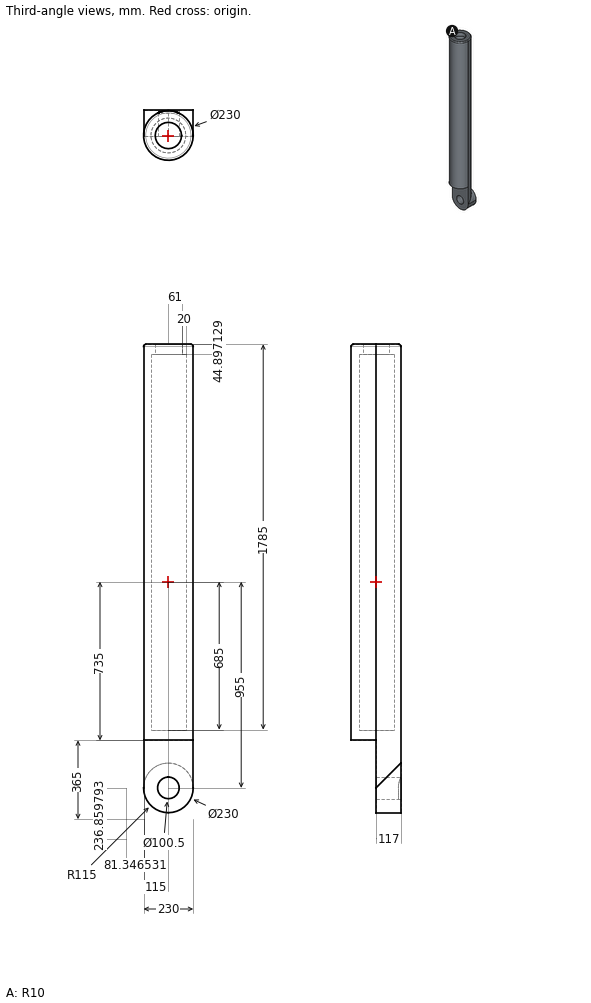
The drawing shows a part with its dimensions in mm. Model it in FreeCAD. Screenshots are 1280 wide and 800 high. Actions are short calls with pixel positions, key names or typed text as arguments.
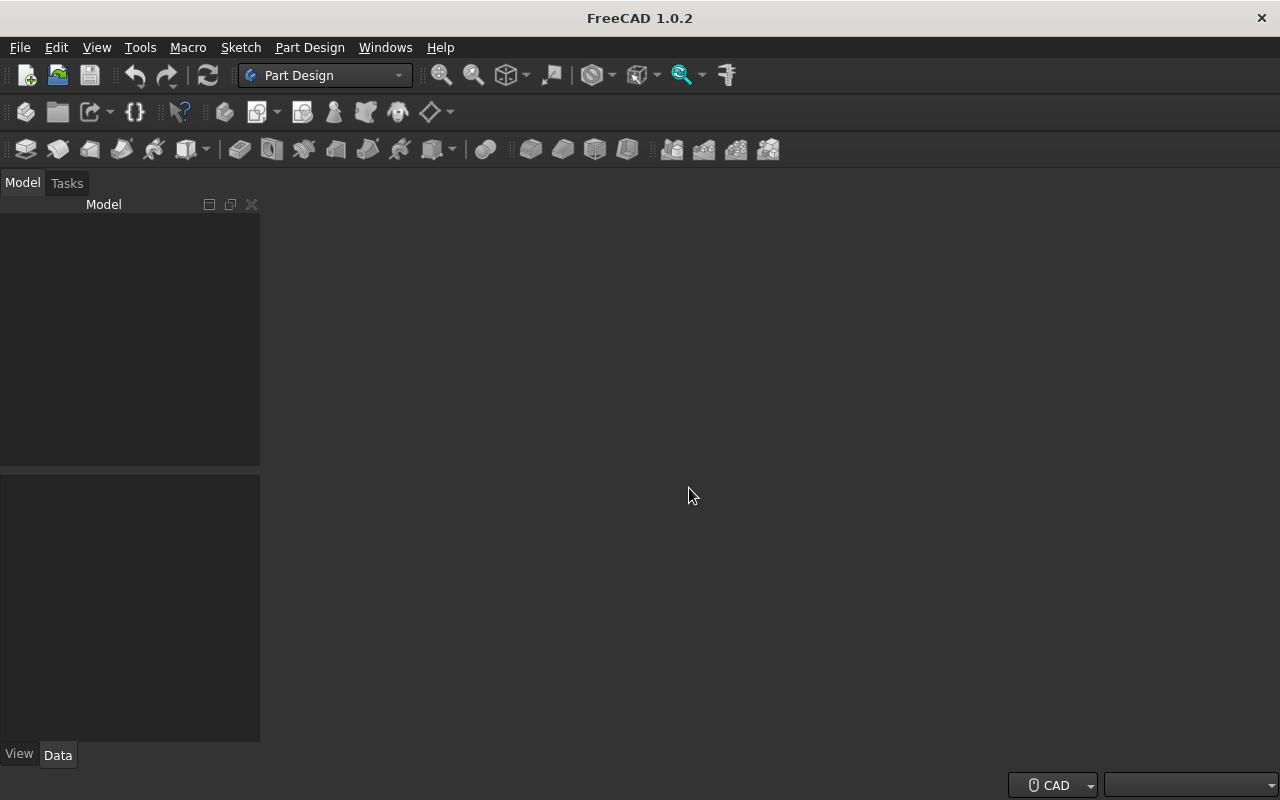
click(26, 76)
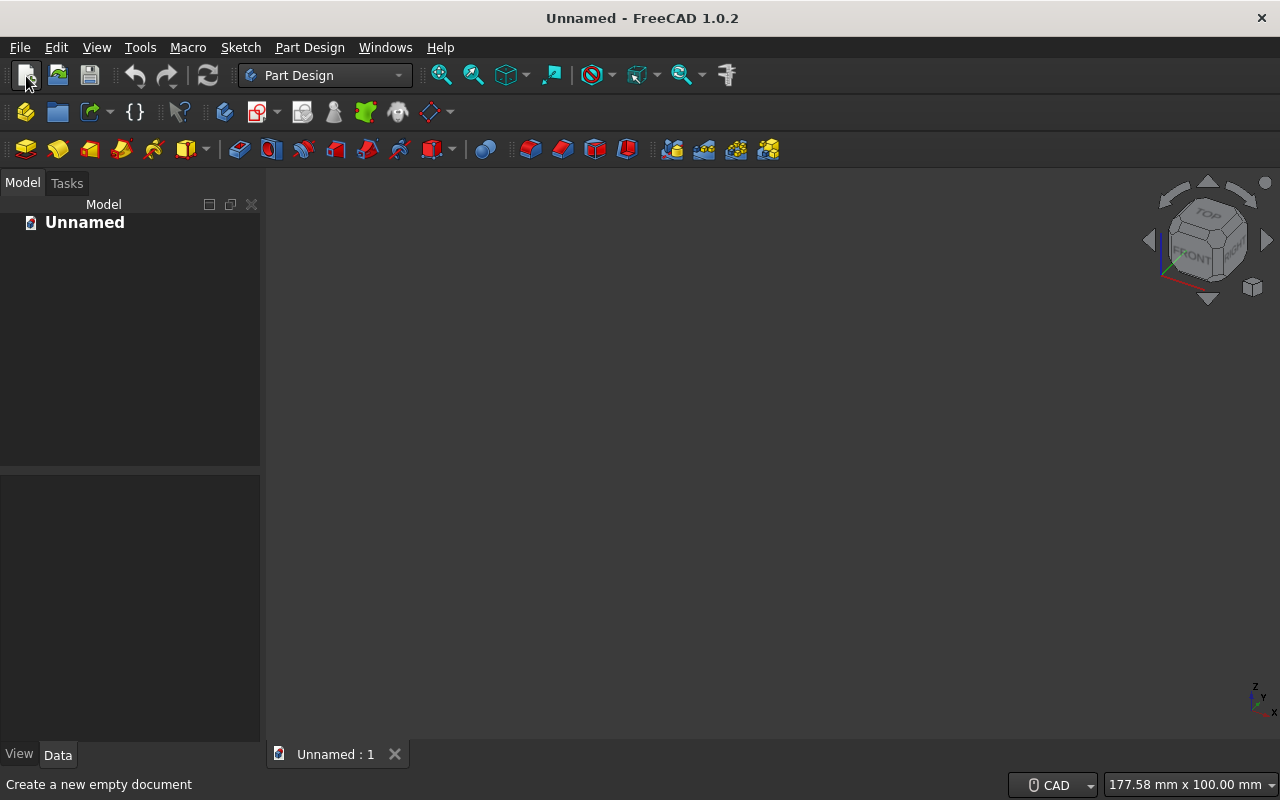
click(258, 112)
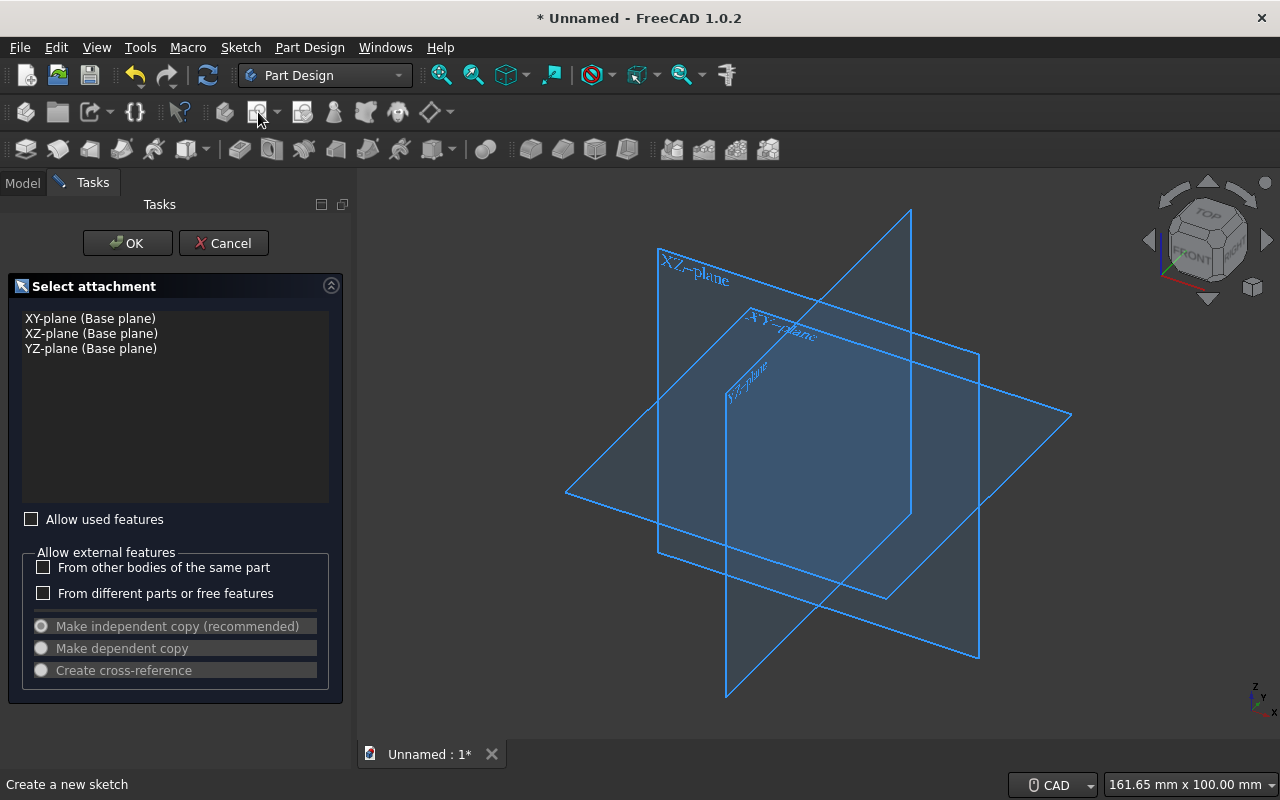
click(82, 318)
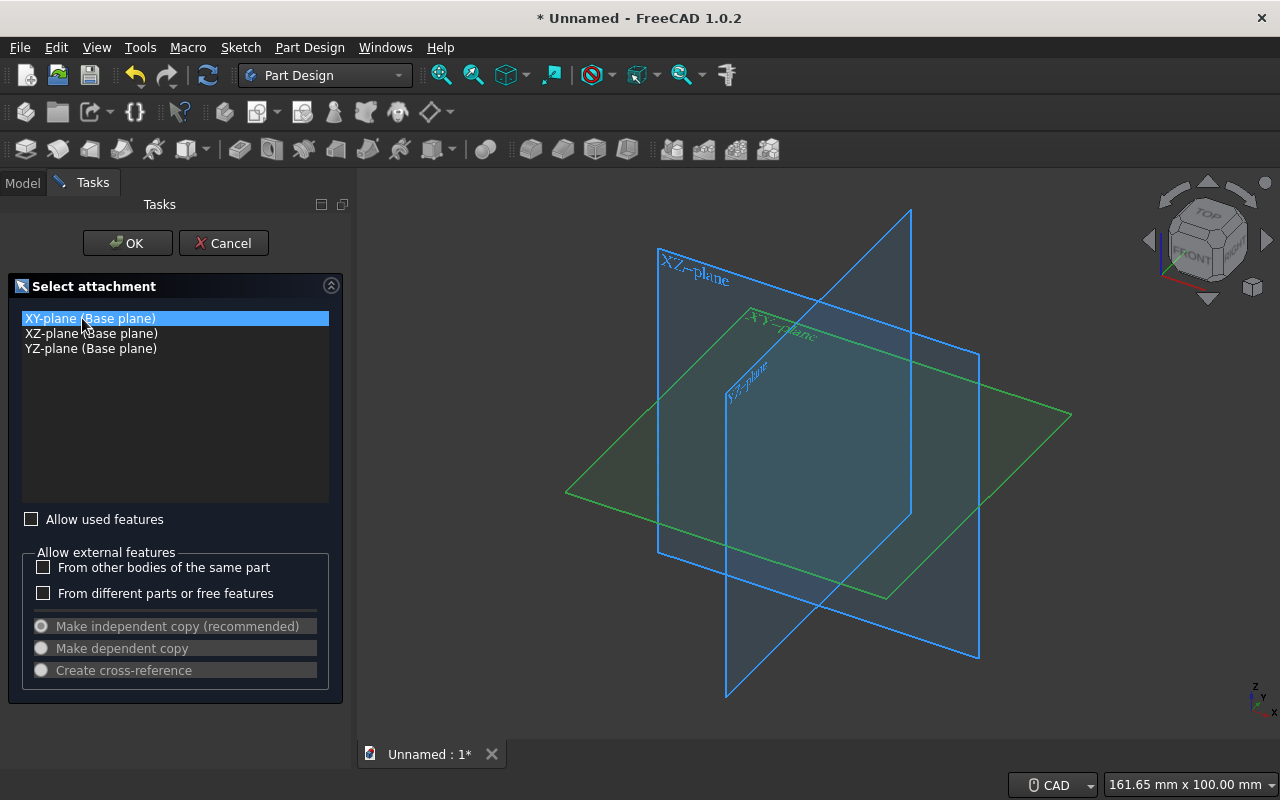
click(128, 243)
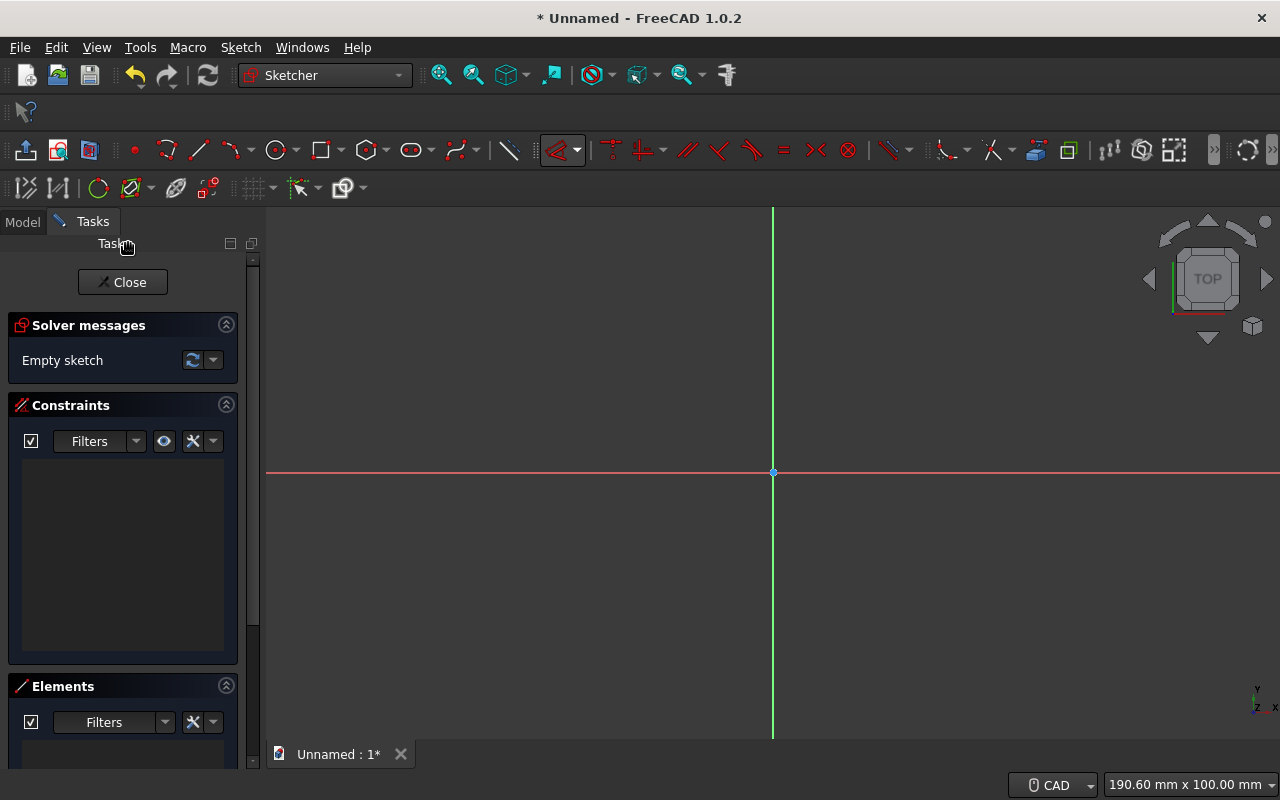
scroll(675, 473, down, 6)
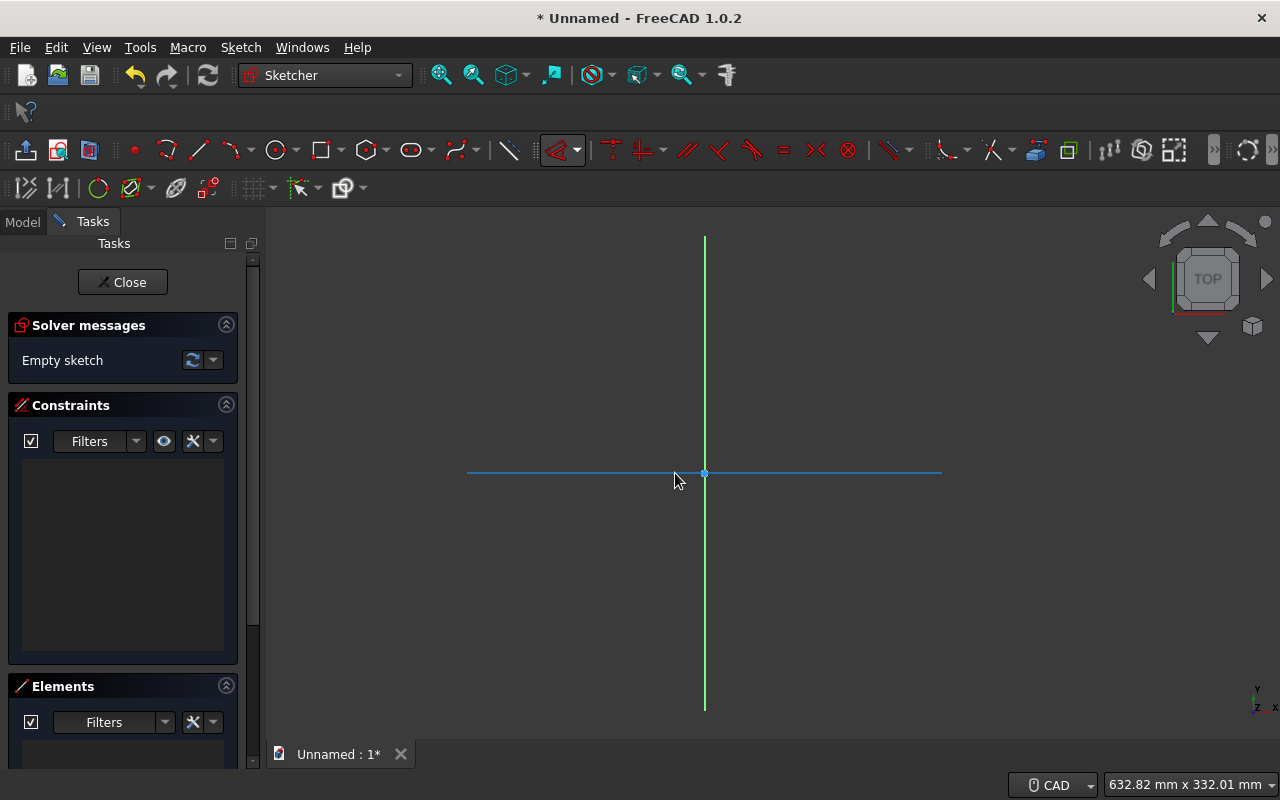
click(276, 150)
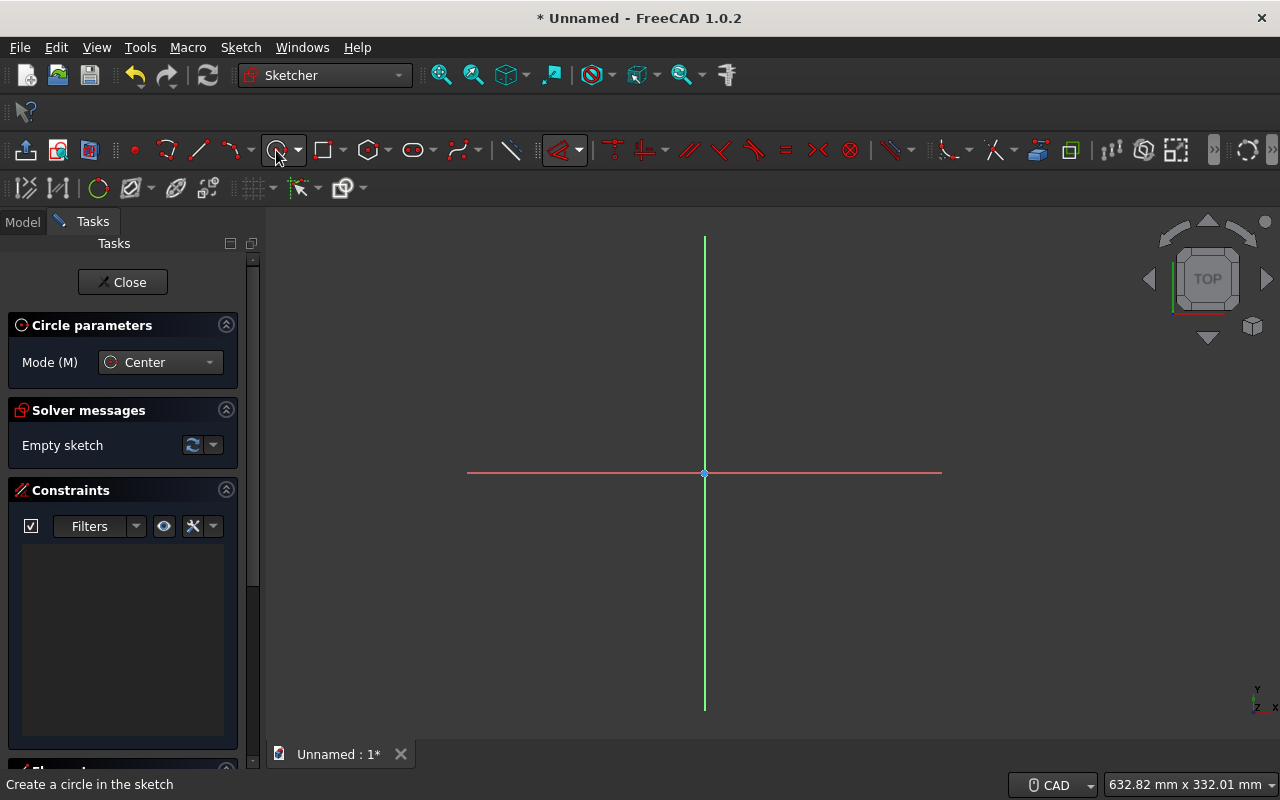
click(705, 473)
click(835, 343)
key(Escape)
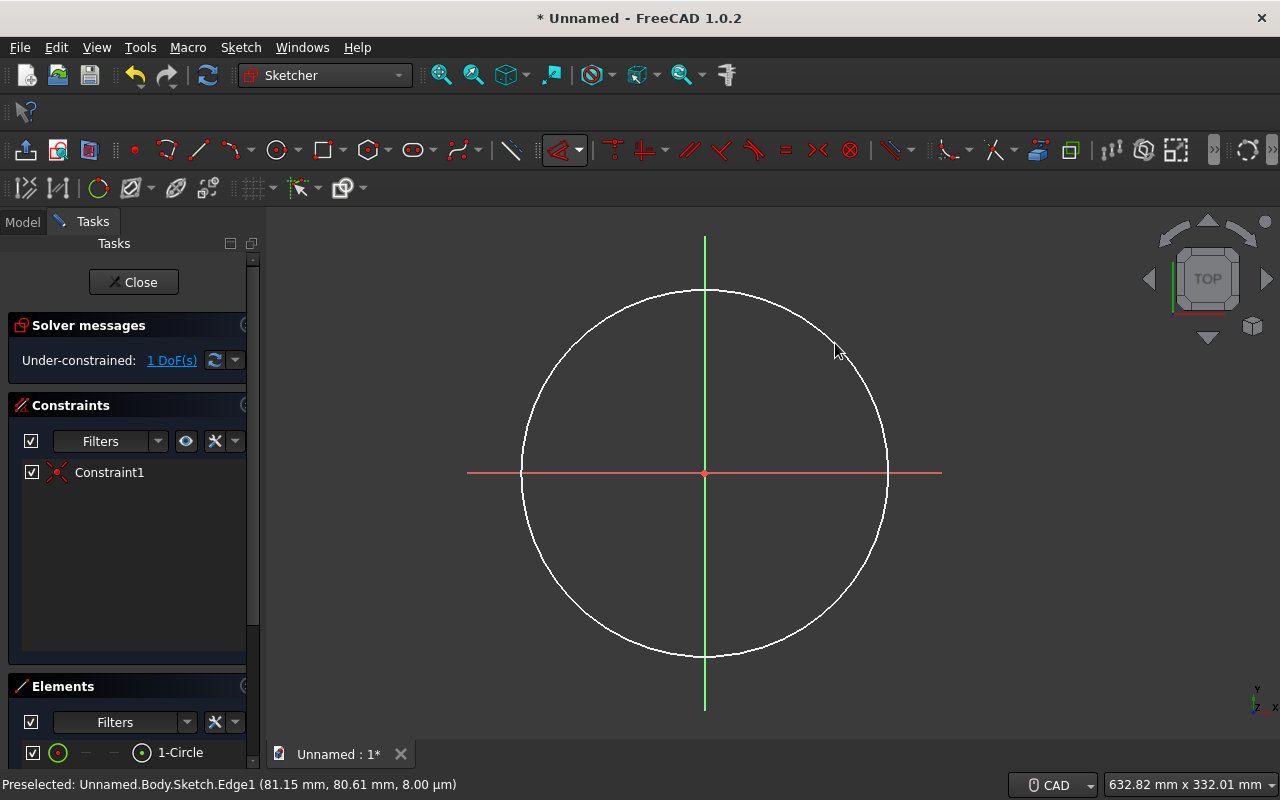
click(558, 150)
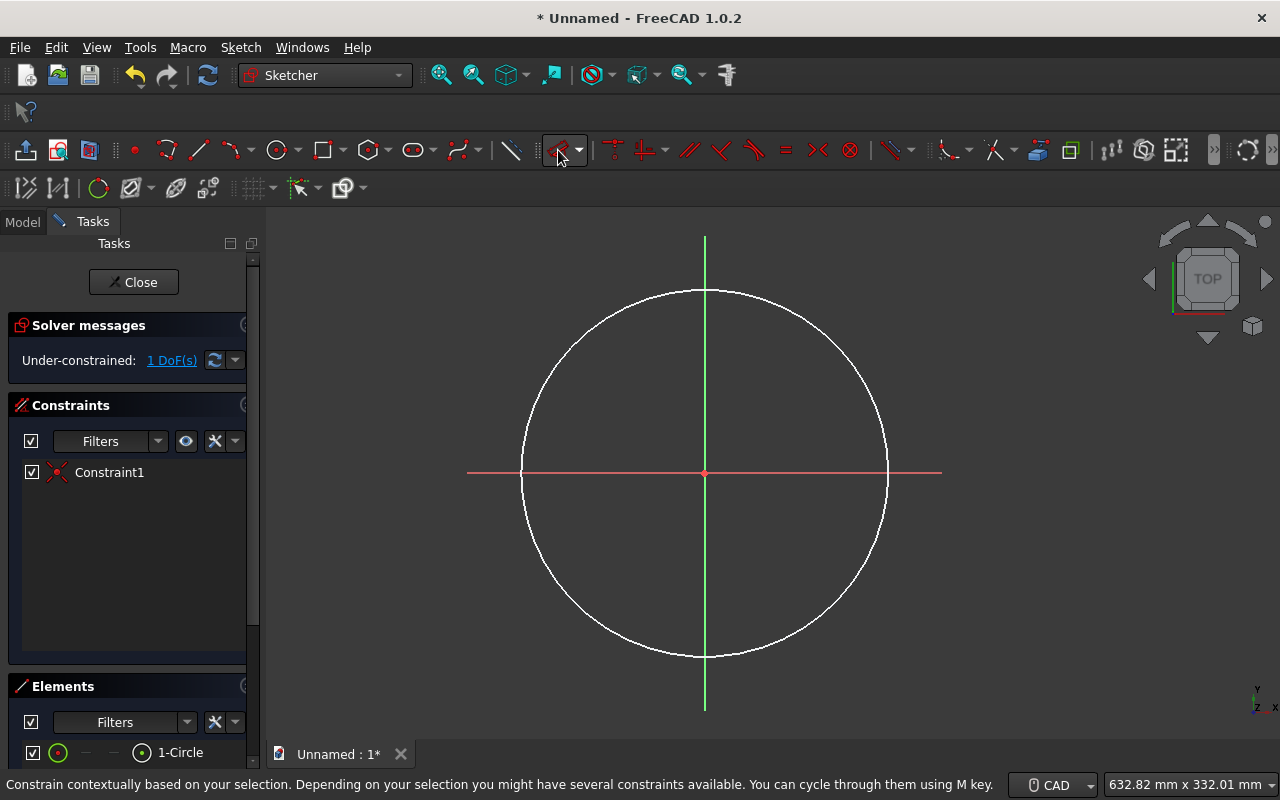
click(834, 343)
click(857, 320)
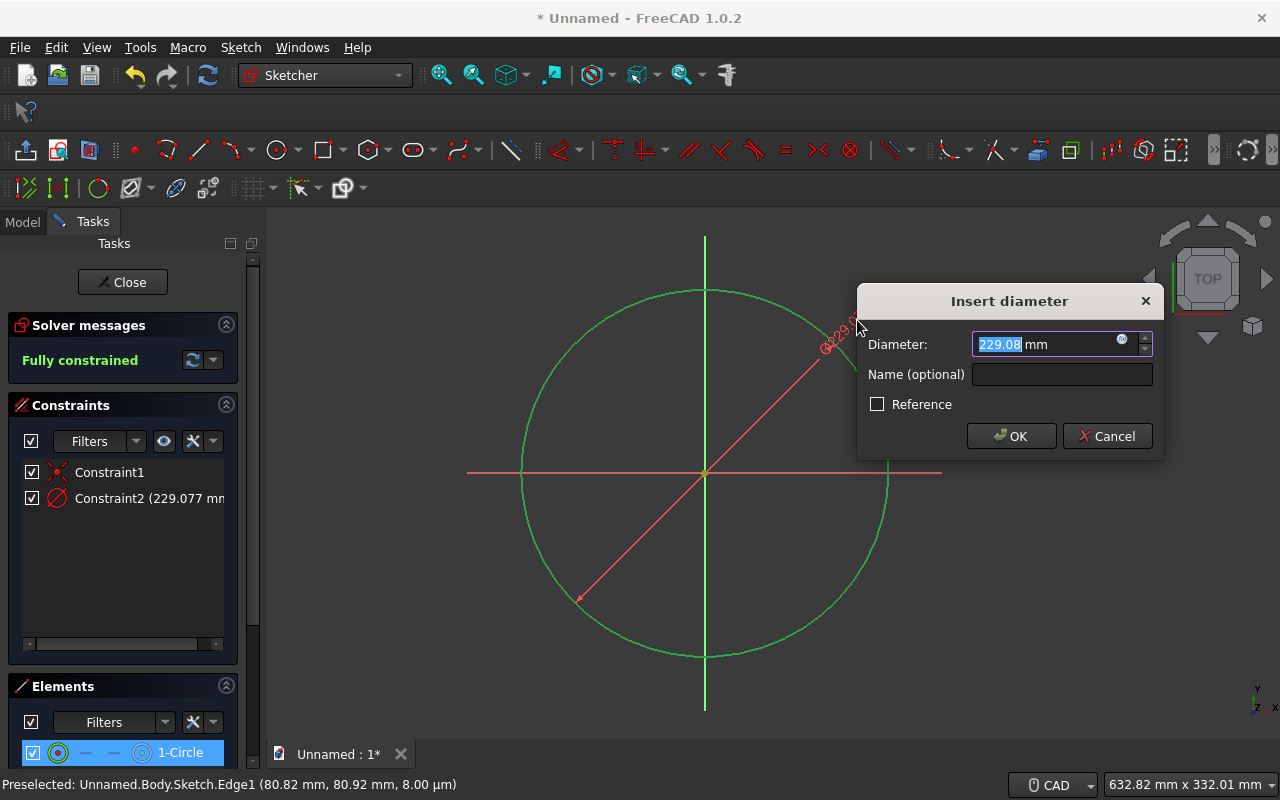
text(230)
key(Return)
key(Escape)